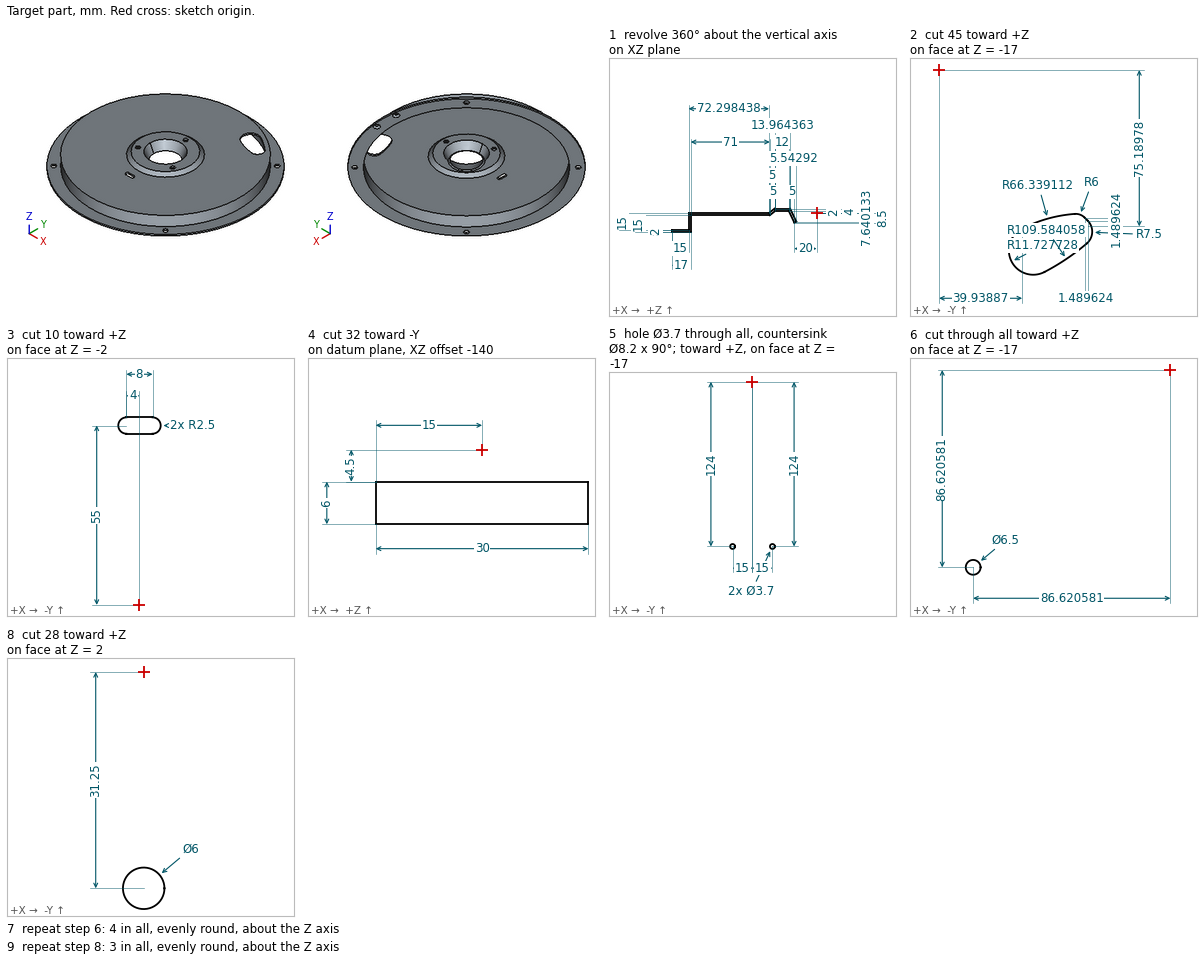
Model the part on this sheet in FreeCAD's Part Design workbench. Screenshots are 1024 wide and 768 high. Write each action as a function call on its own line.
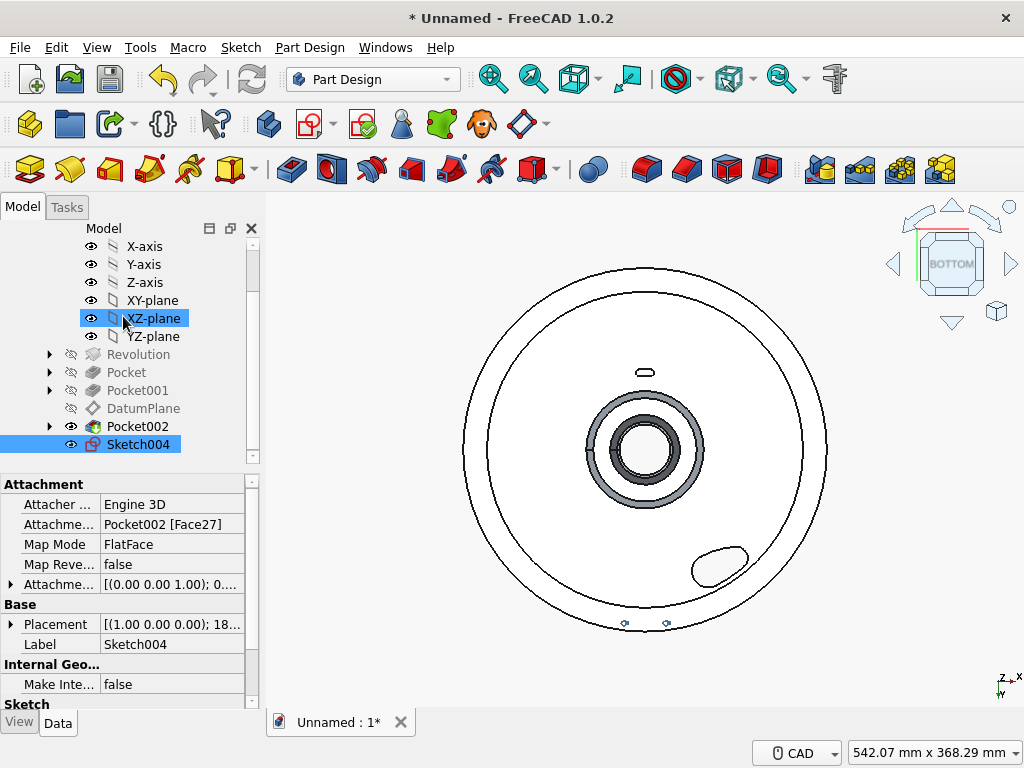
click(332, 170)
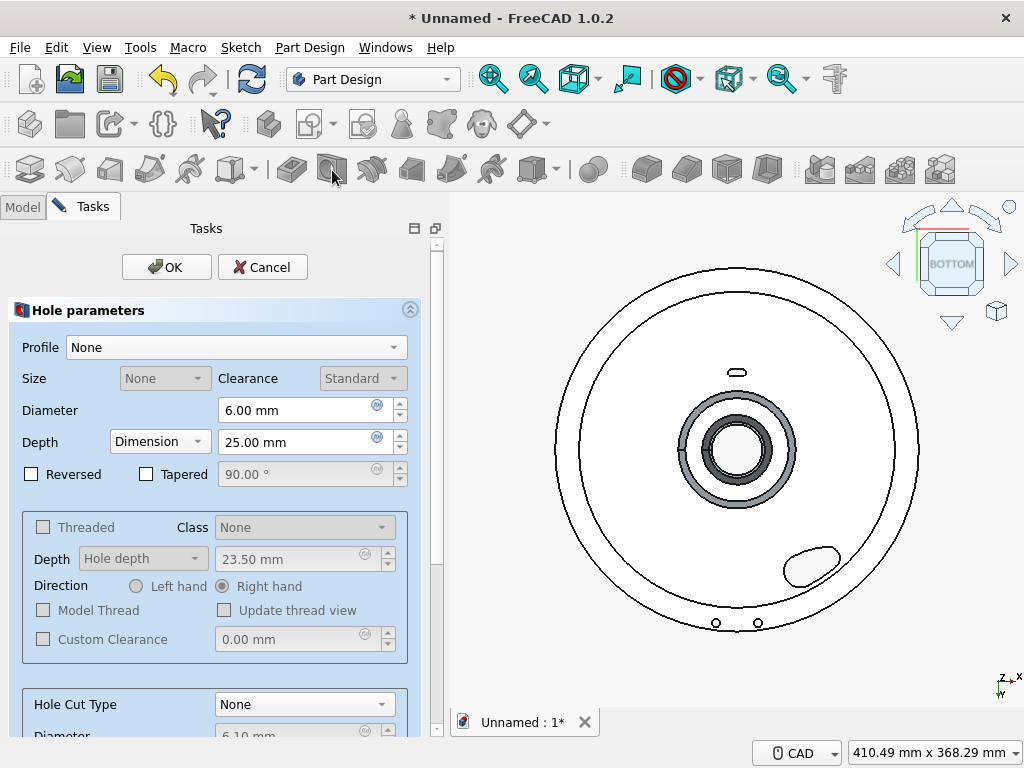
triple_click(305, 410)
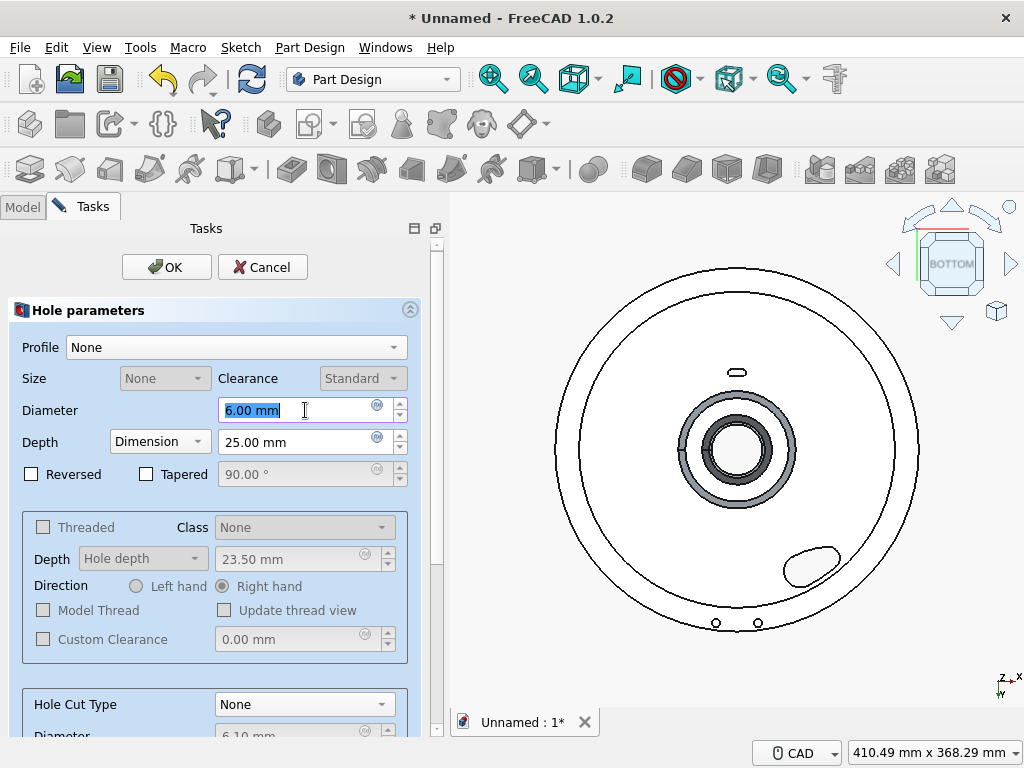
text(3.7)
key(Tab)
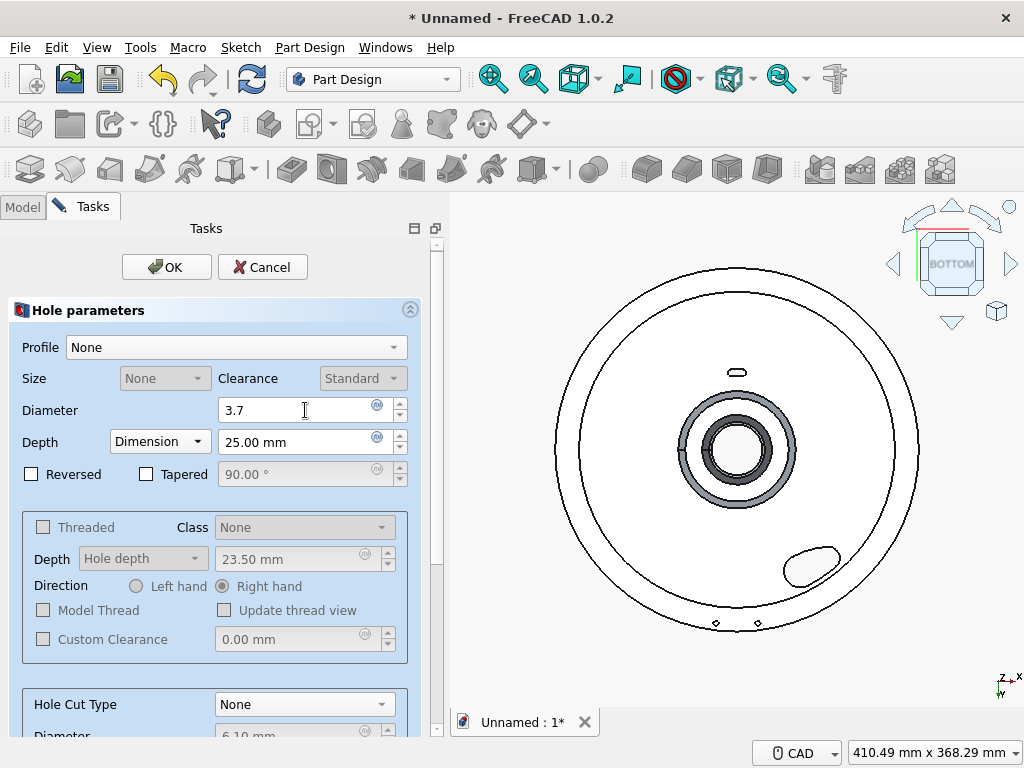
click(161, 442)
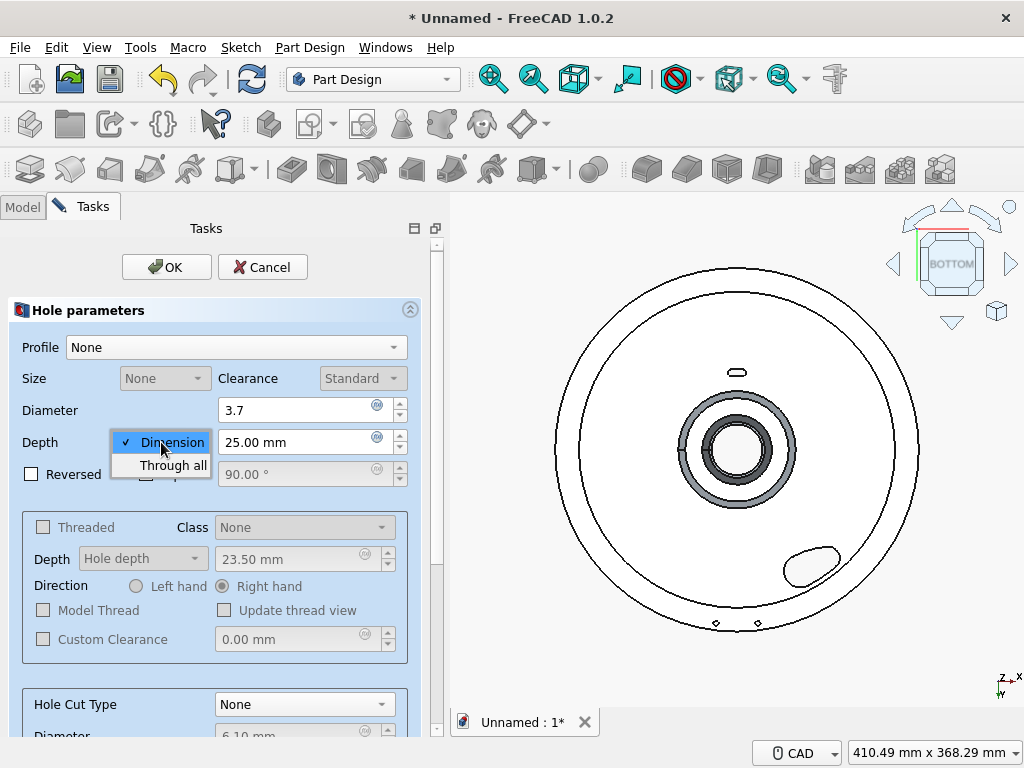
click(160, 466)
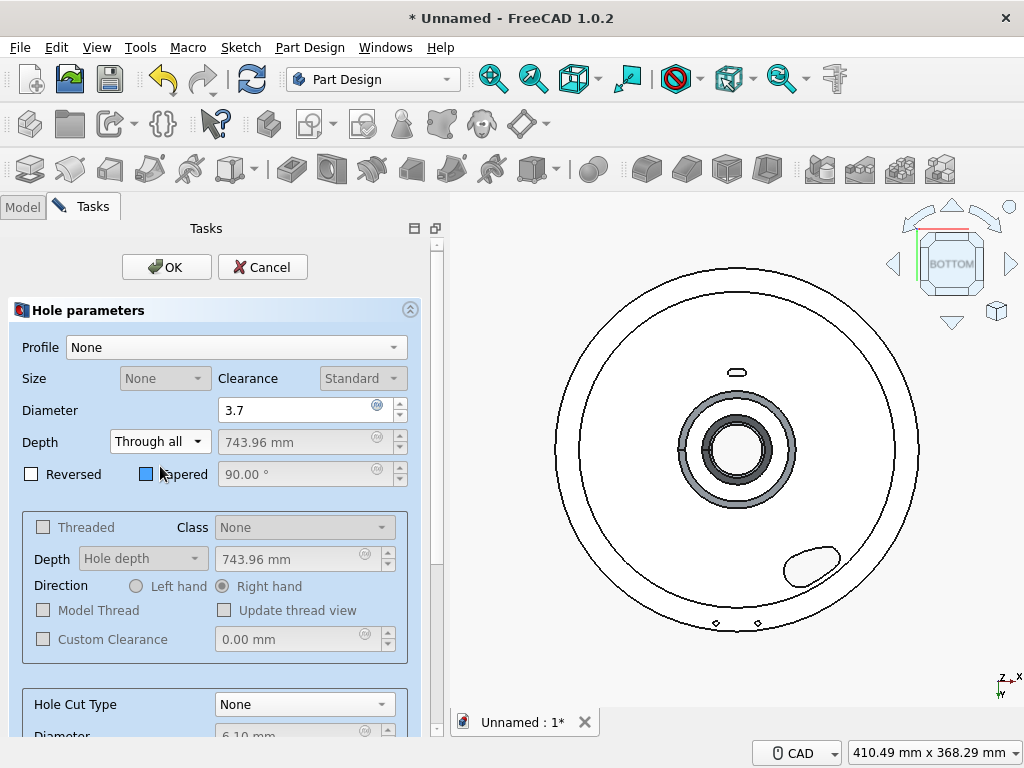
click(306, 704)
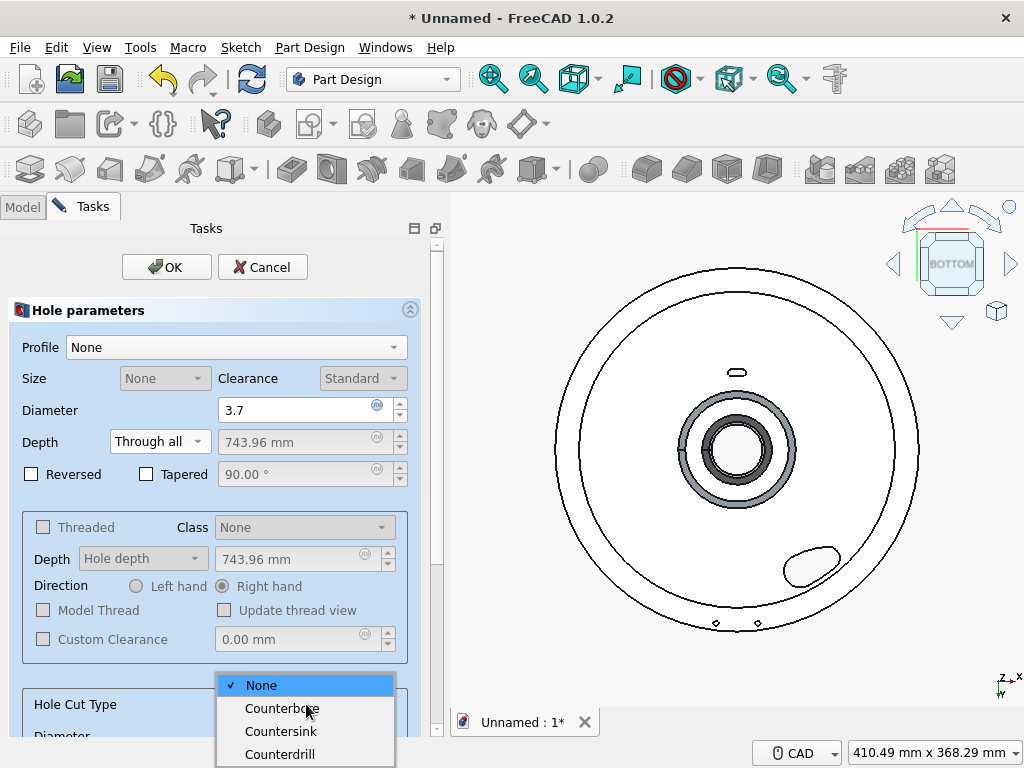
click(304, 732)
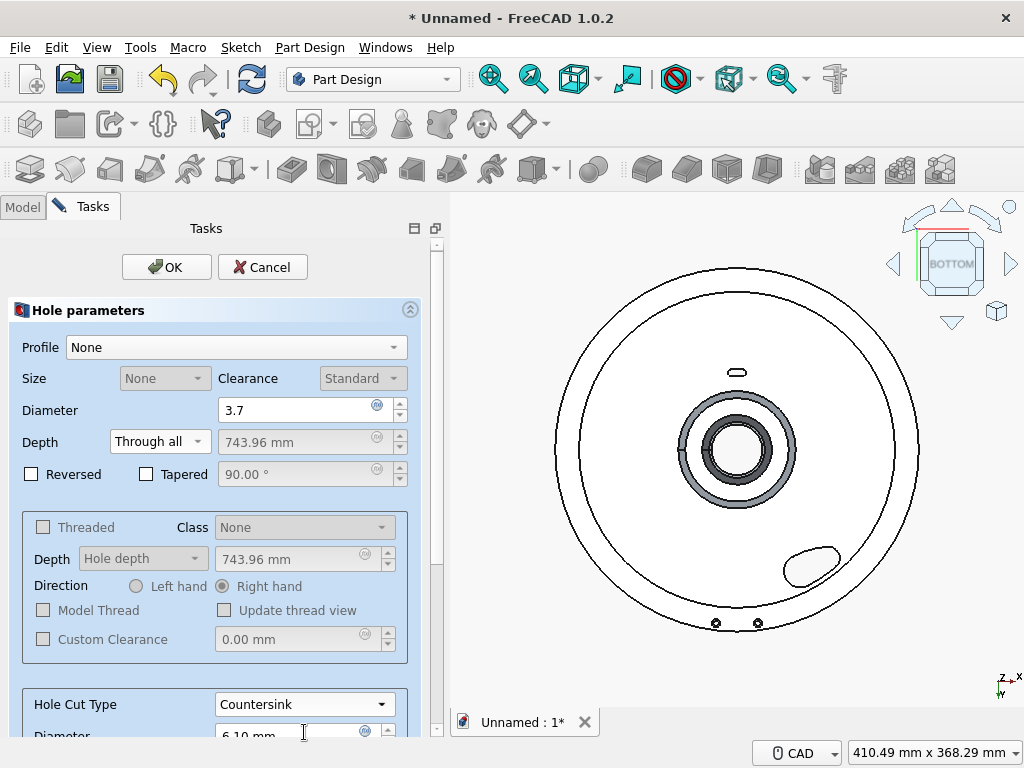
scroll(437, 487, down, 2)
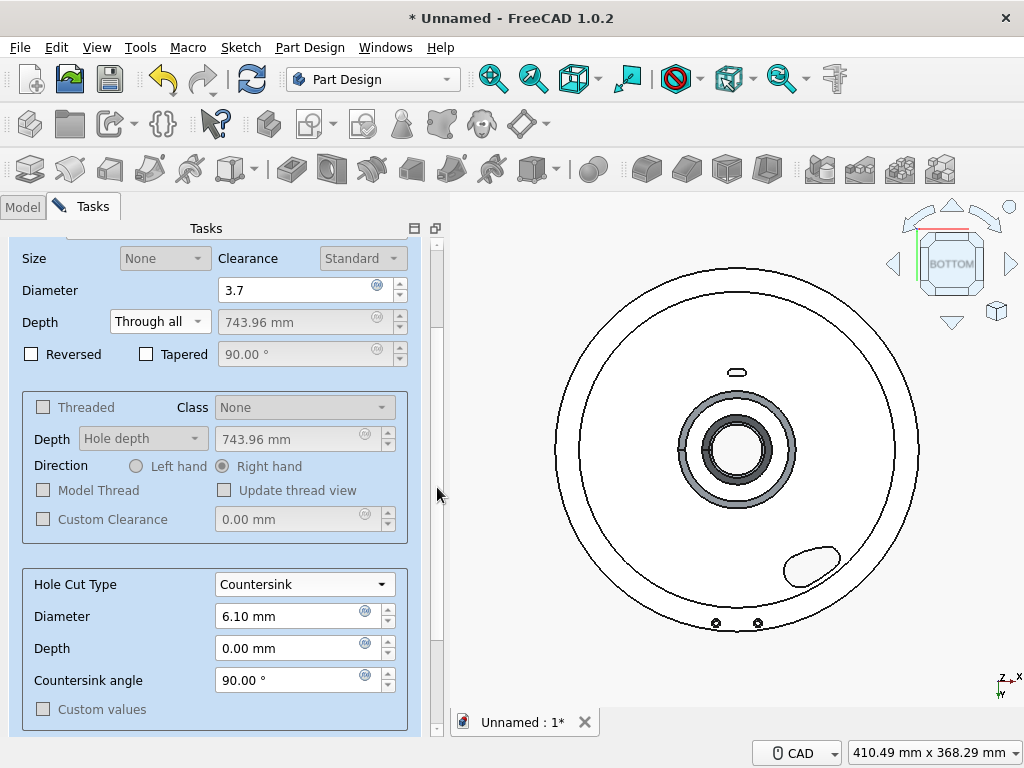
triple_click(298, 616)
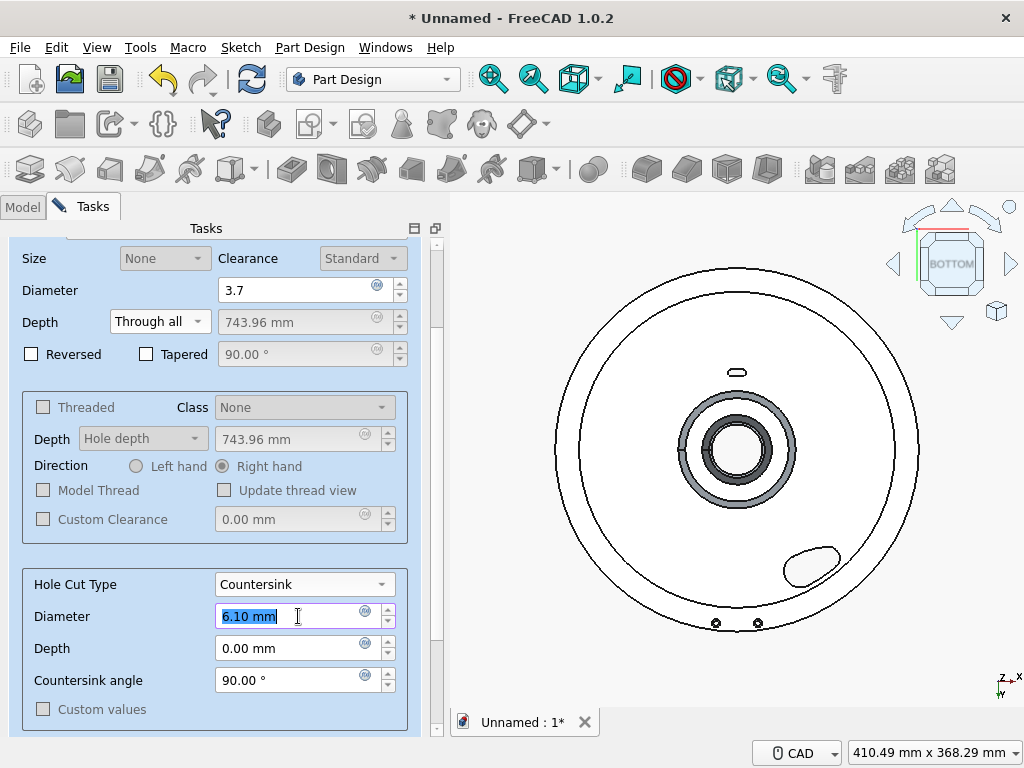
text(8.2)
key(Tab)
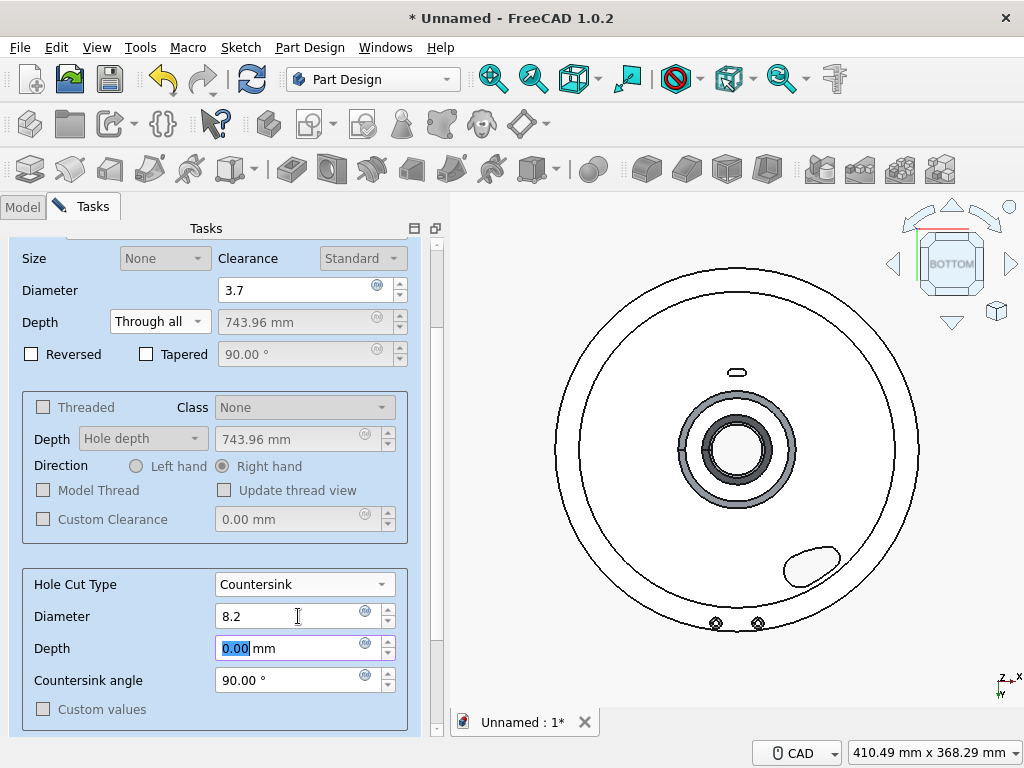
scroll(437, 487, up, 3)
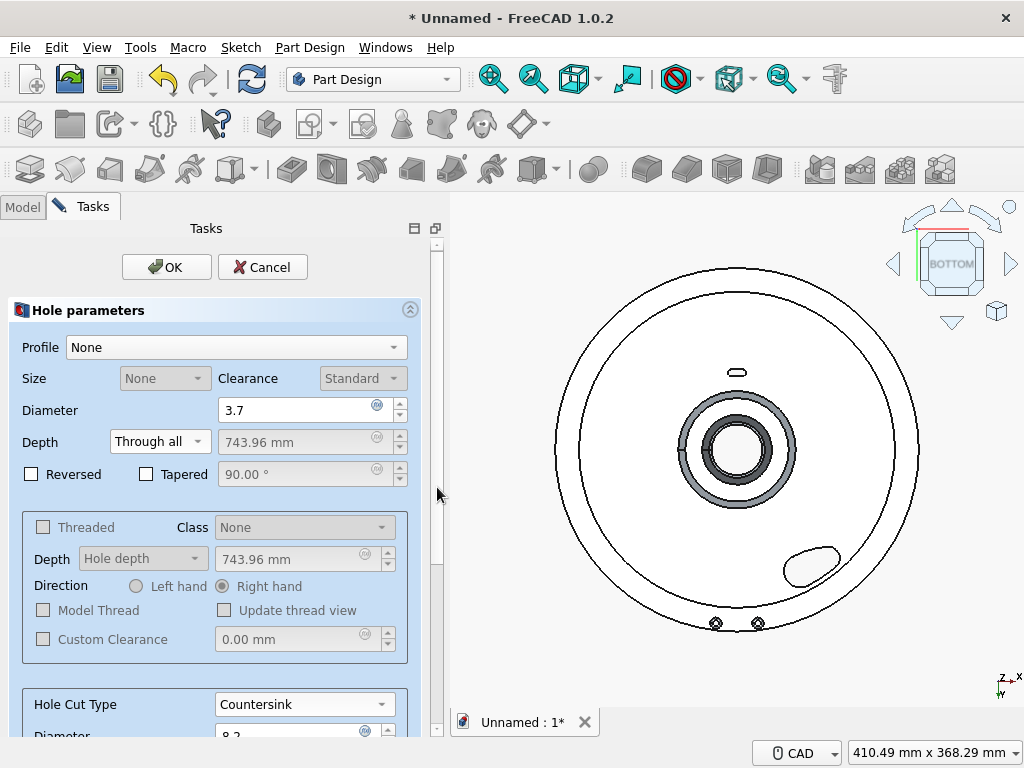
click(167, 267)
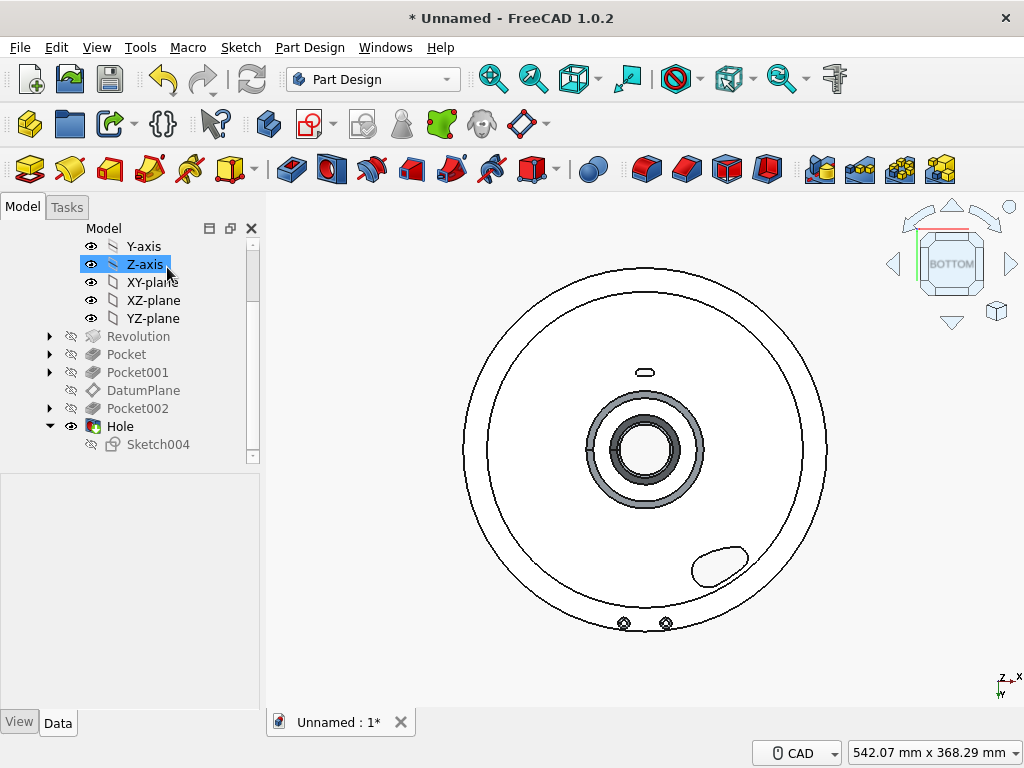
click(593, 293)